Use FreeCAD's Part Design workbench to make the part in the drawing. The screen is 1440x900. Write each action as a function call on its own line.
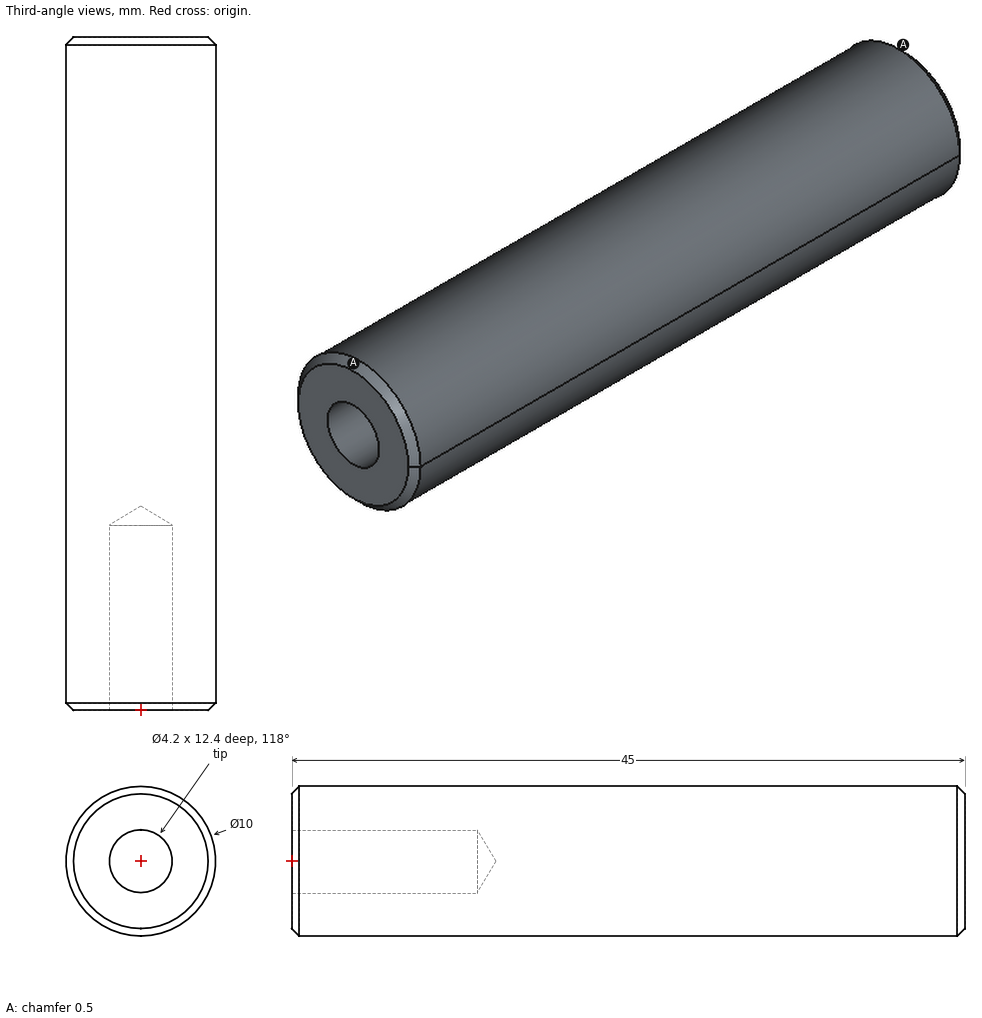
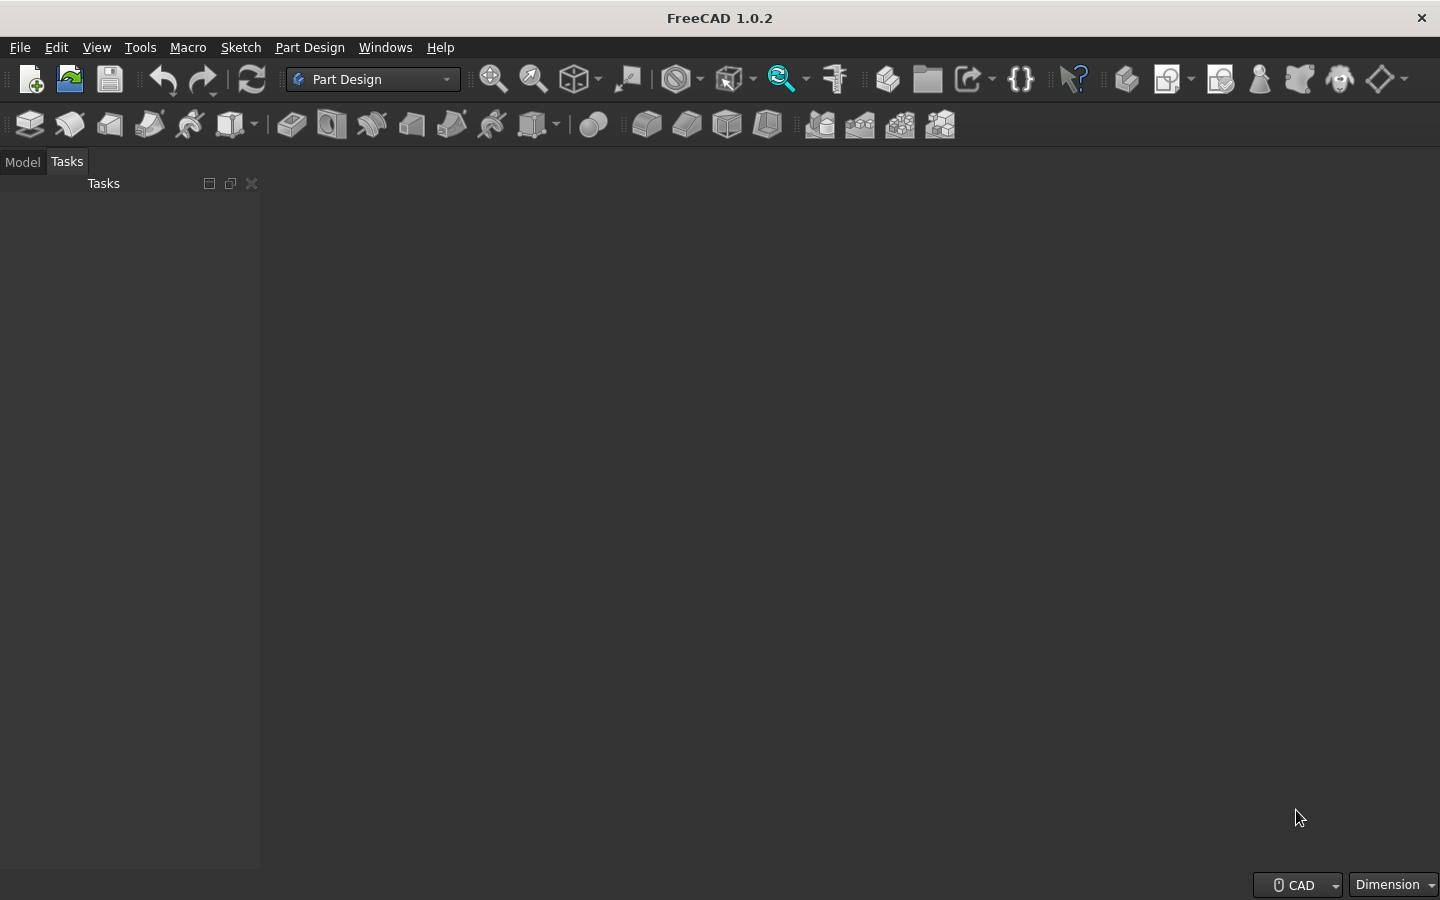
click(30, 80)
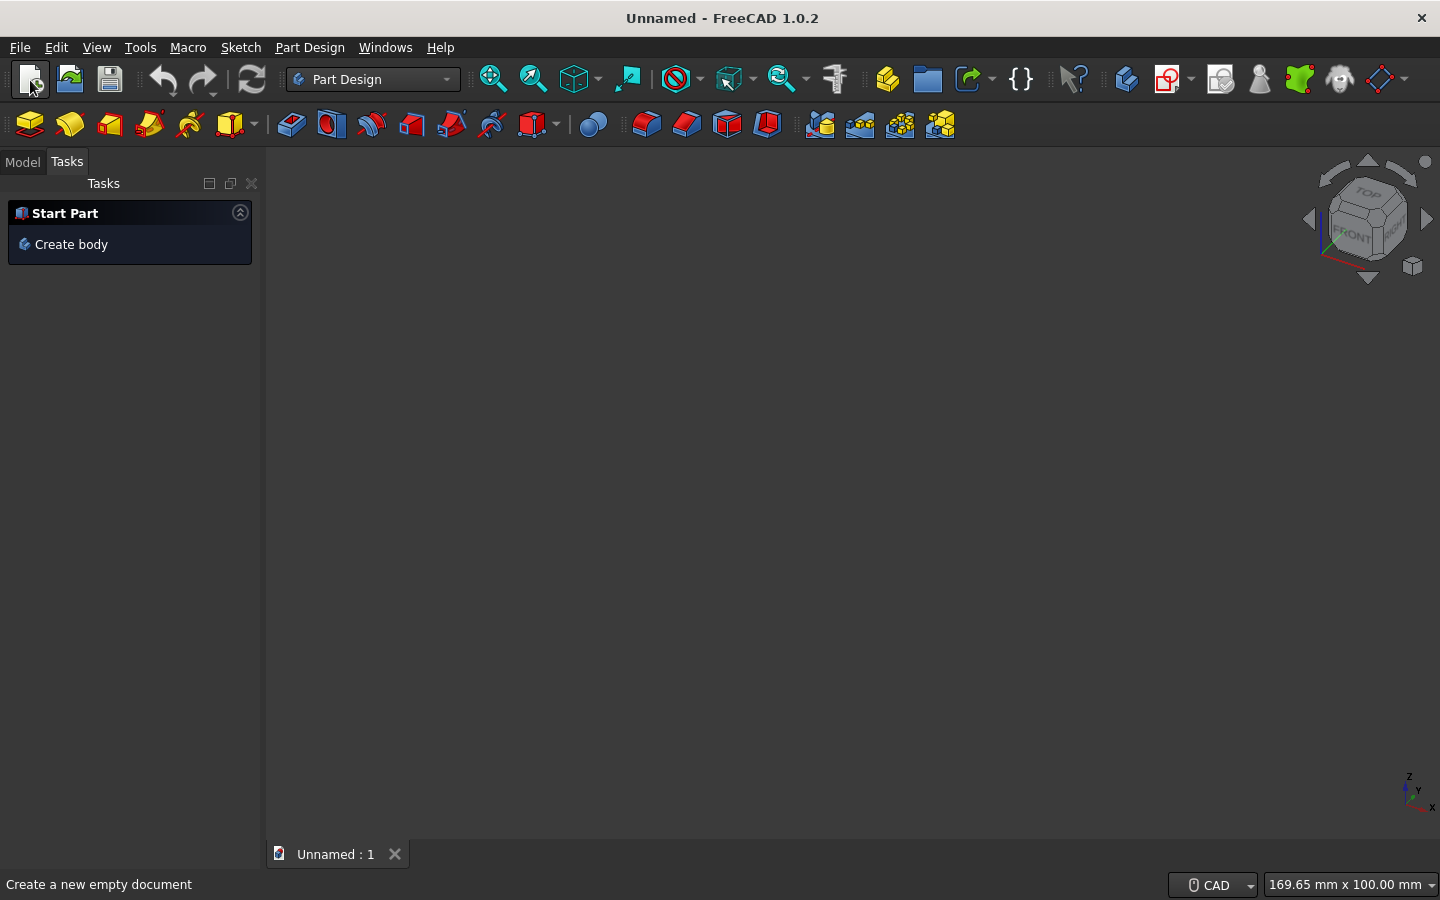
click(1168, 80)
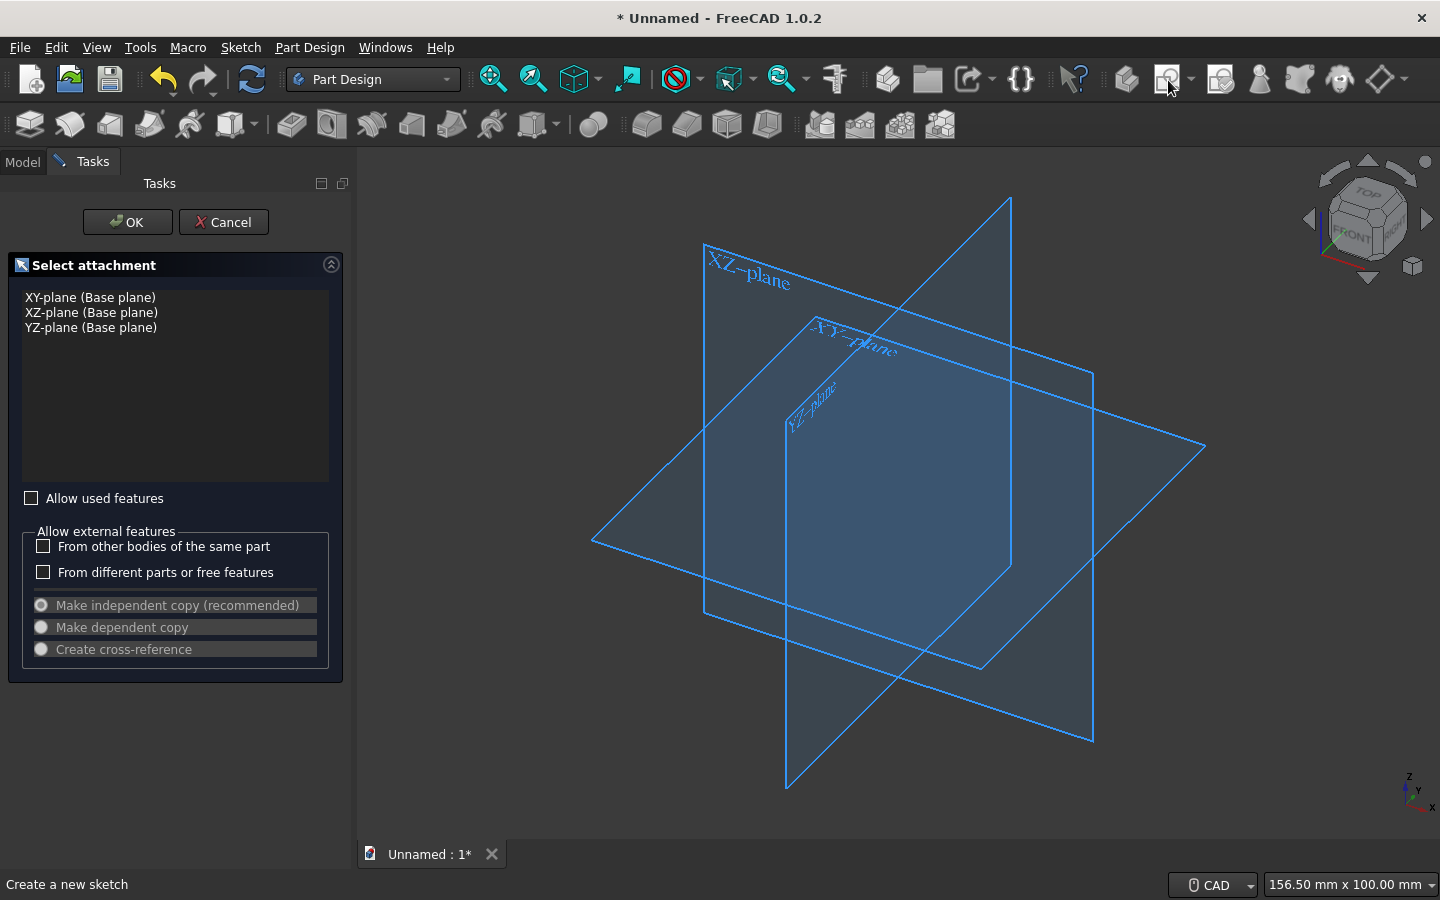
click(82, 312)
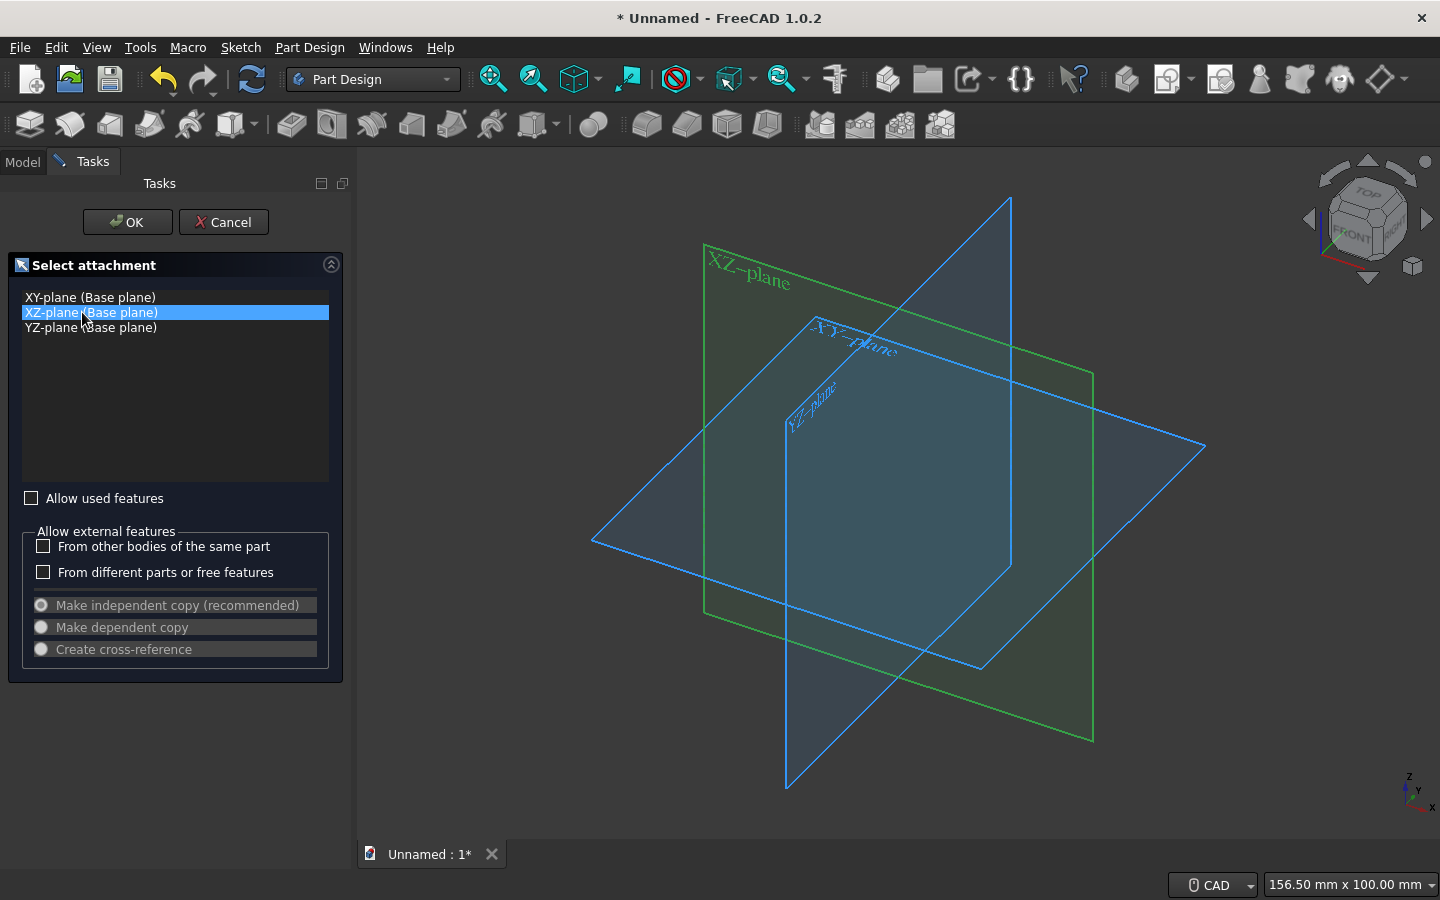
click(128, 222)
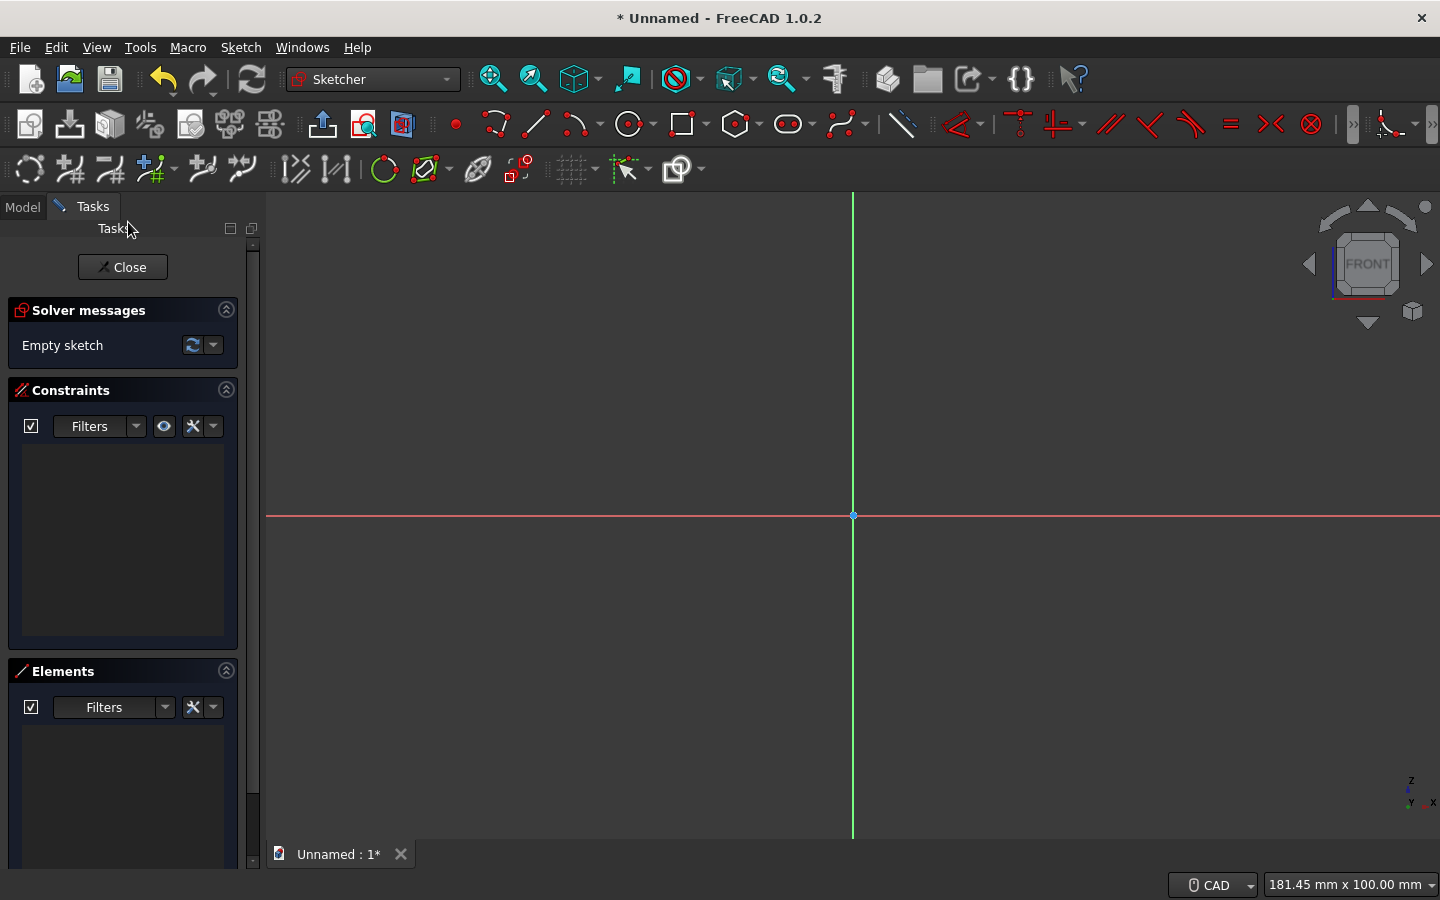
scroll(867, 516, up, 9)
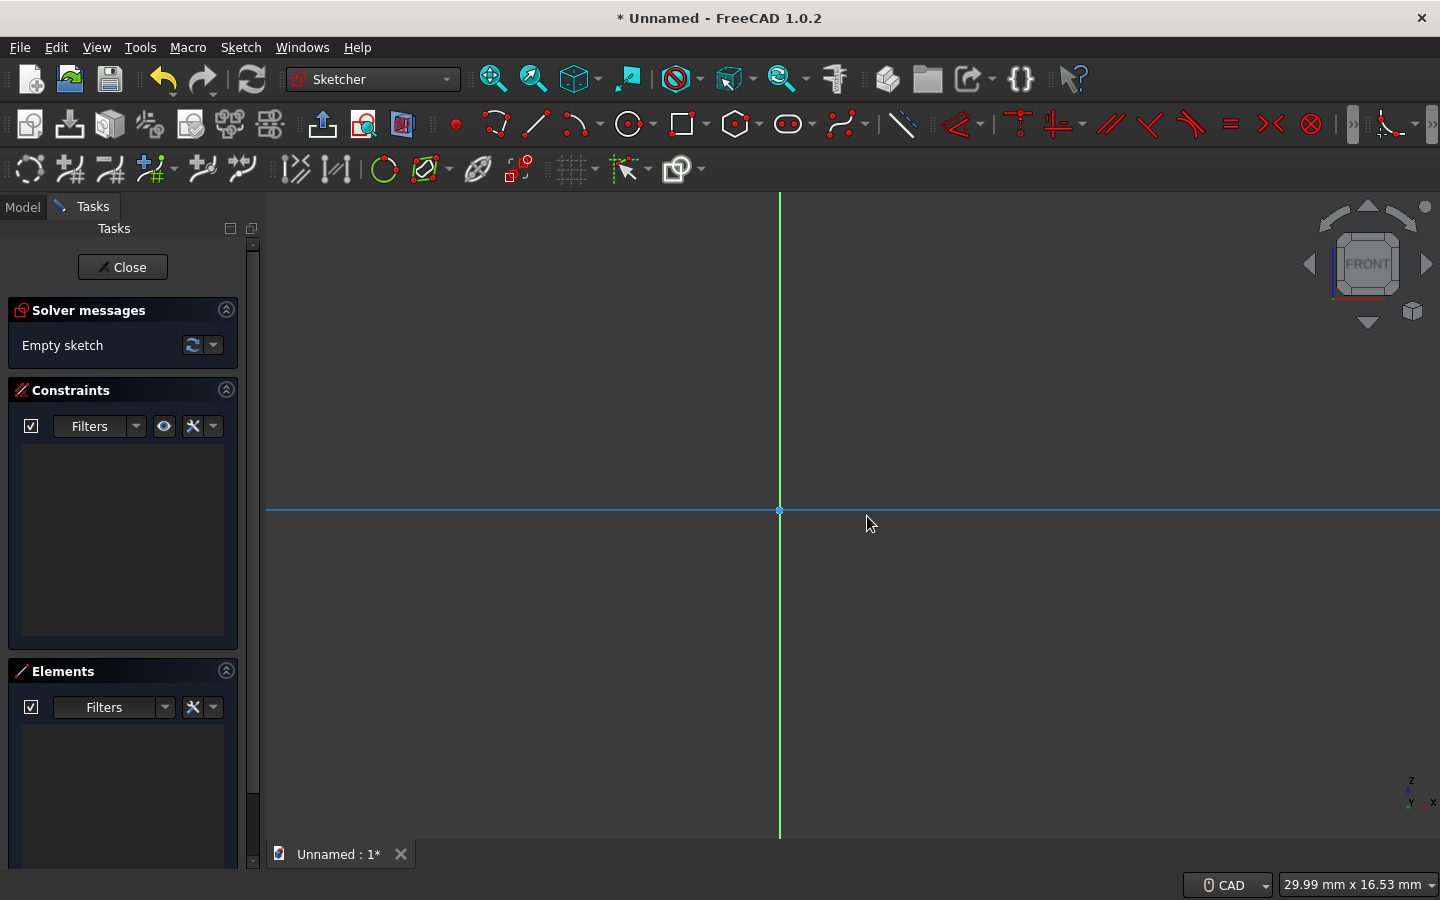
click(630, 124)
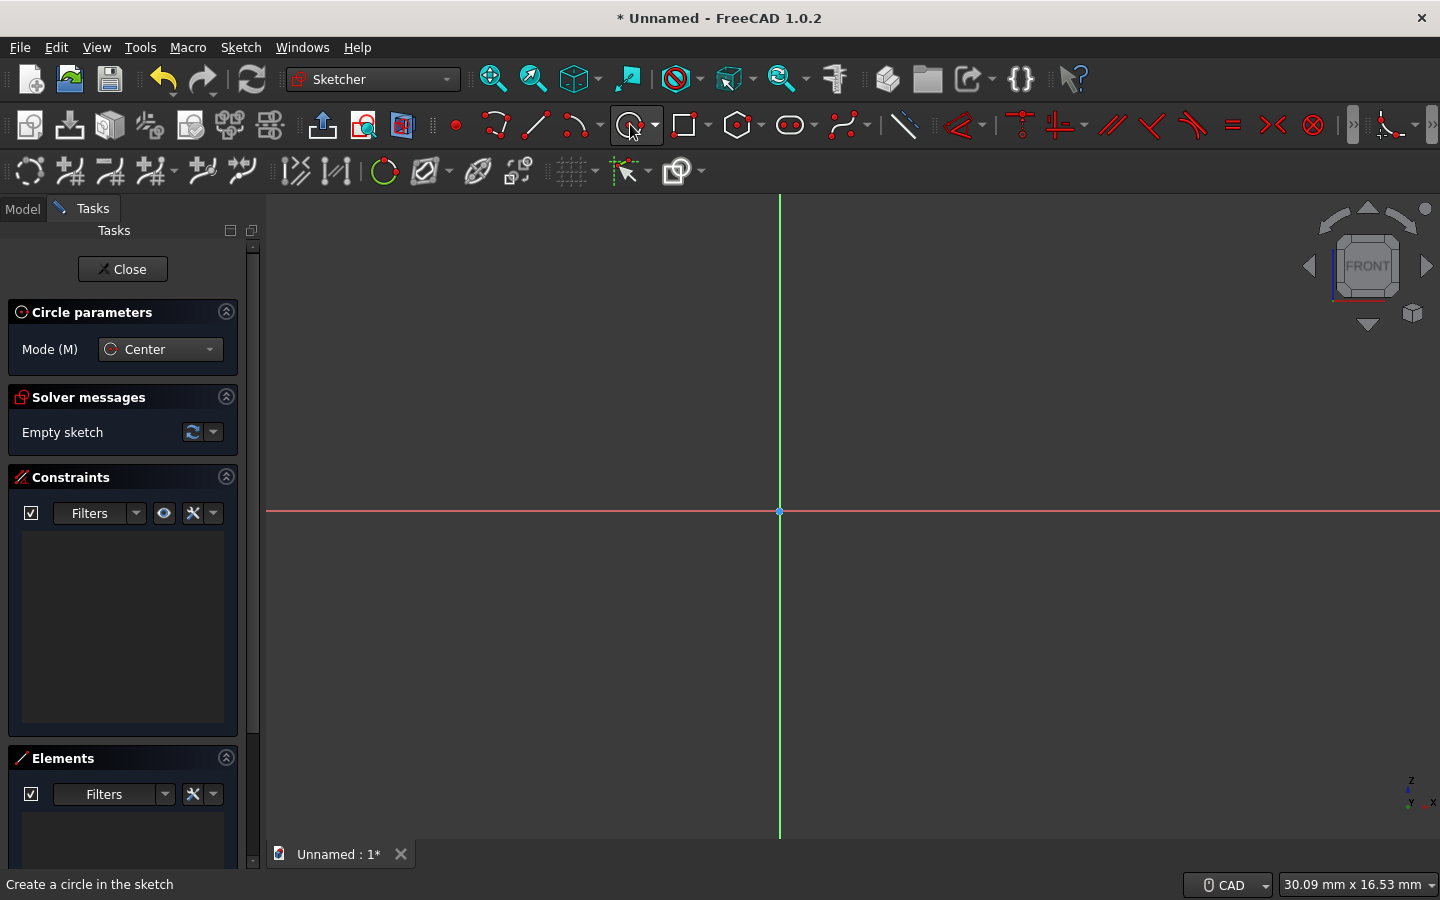
click(780, 511)
move(918, 374)